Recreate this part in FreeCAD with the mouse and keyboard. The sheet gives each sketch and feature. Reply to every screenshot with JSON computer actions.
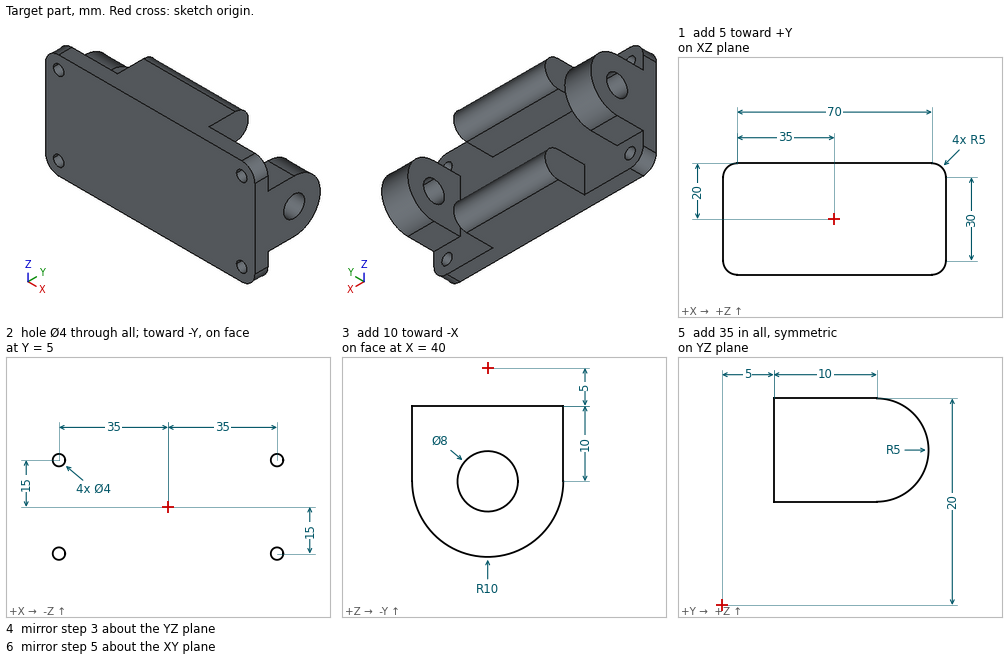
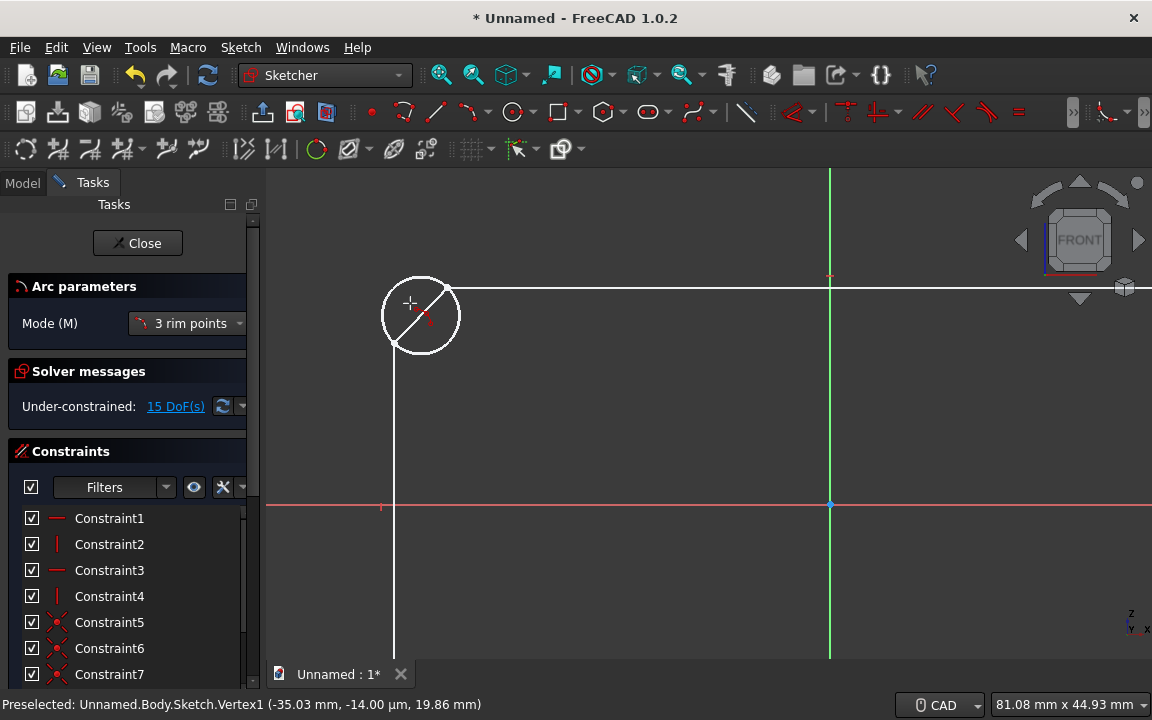
{"action": "left_click", "coordinate": [409, 302]}
{"action": "key", "text": "Escape"}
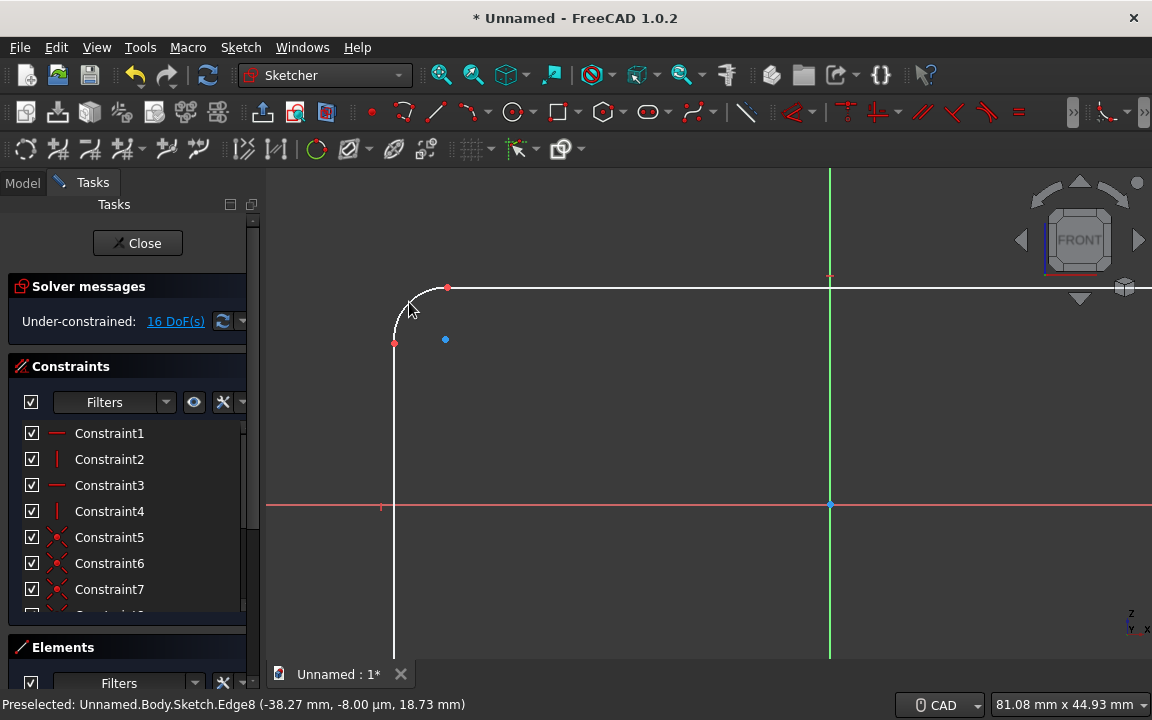
{"action": "left_click", "coordinate": [677, 288]}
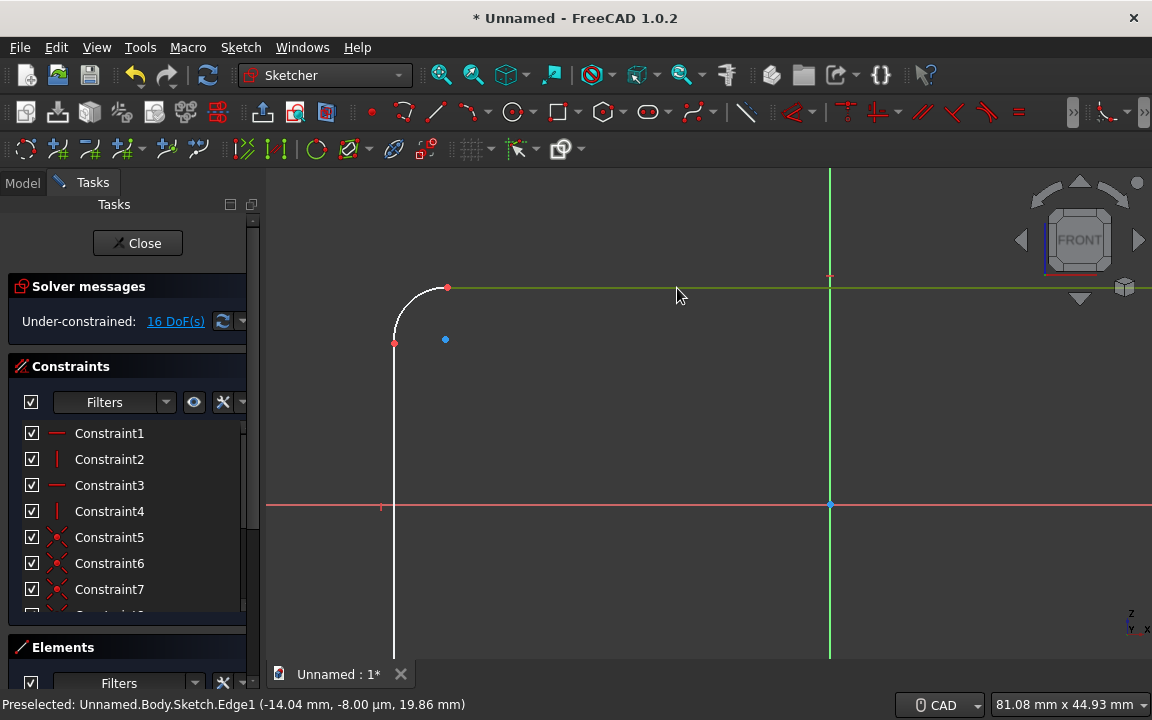
{"action": "scroll", "coordinate": [410, 303], "scroll_direction": "down", "scroll_amount": 3}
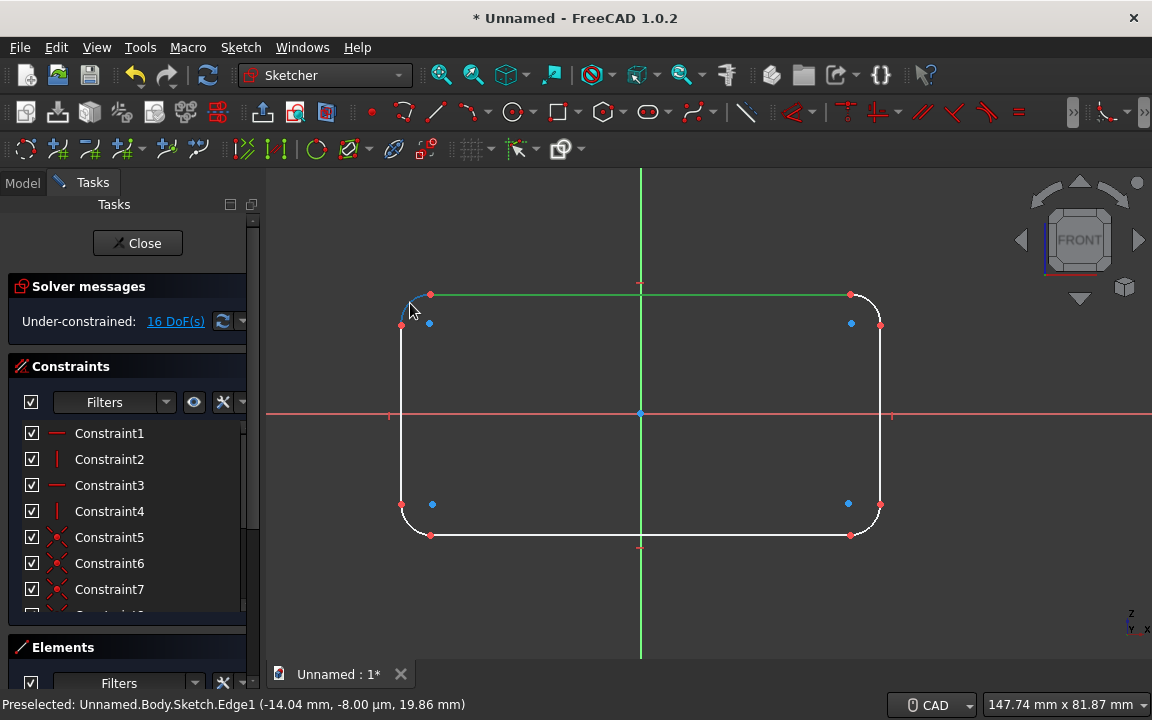
{"action": "left_click", "coordinate": [878, 311]}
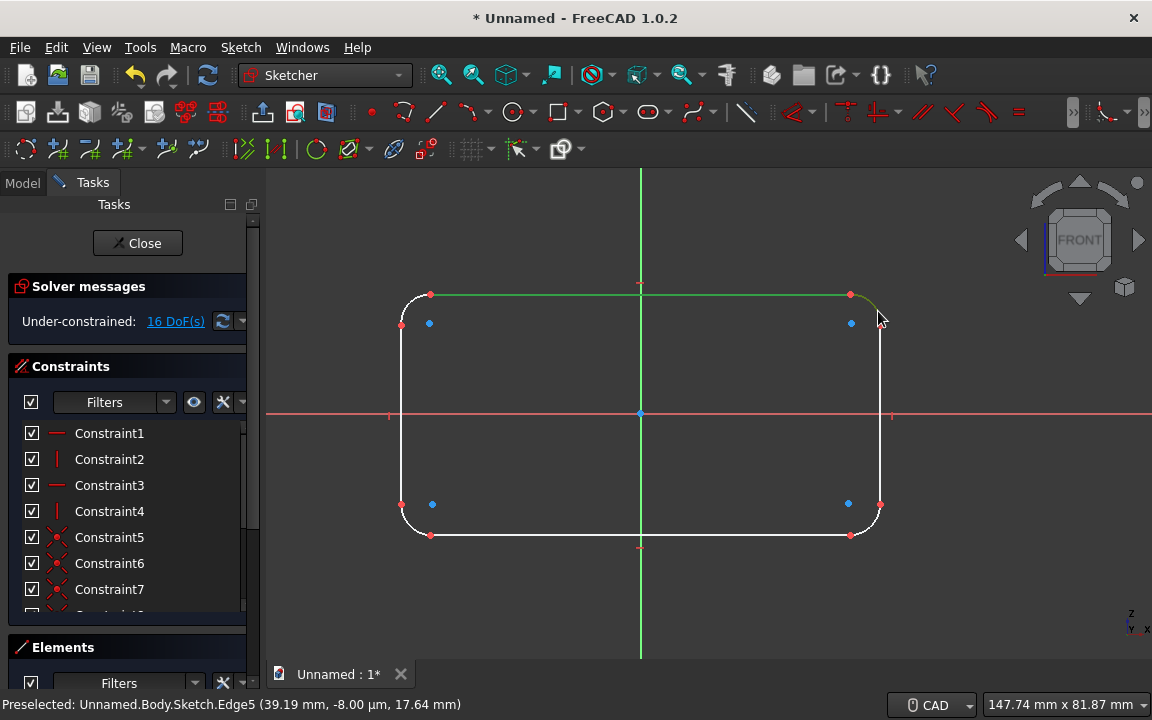
{"action": "key", "text": "t"}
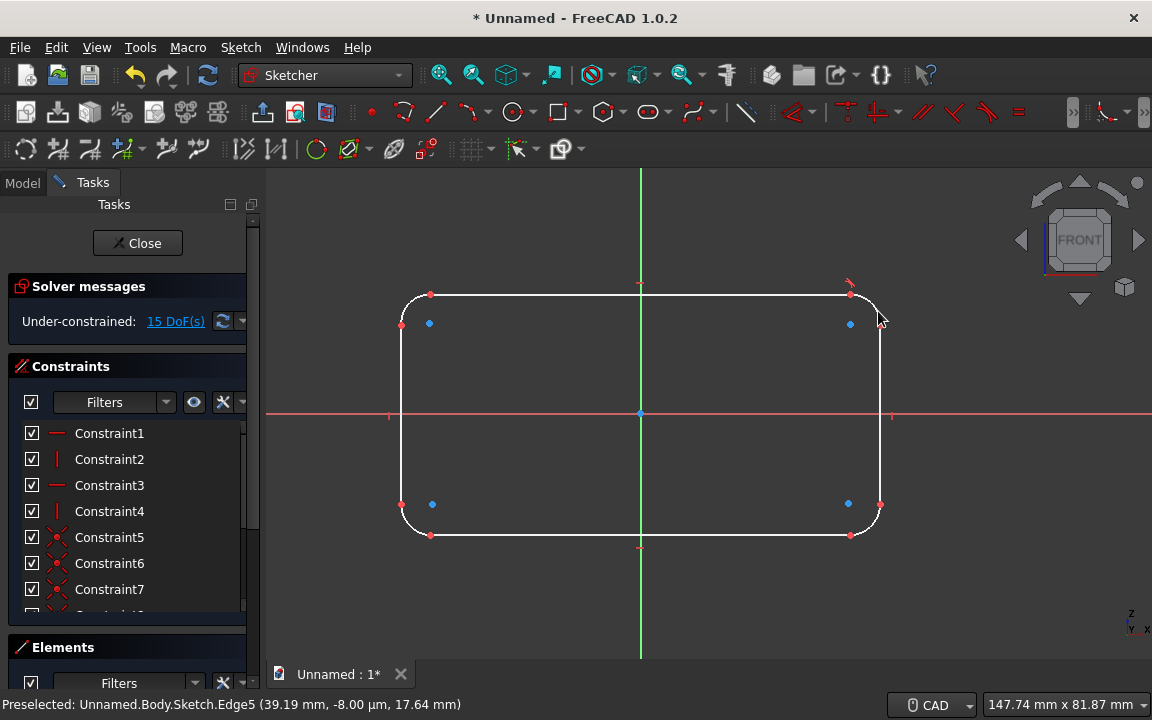
{"action": "left_click", "coordinate": [557, 295]}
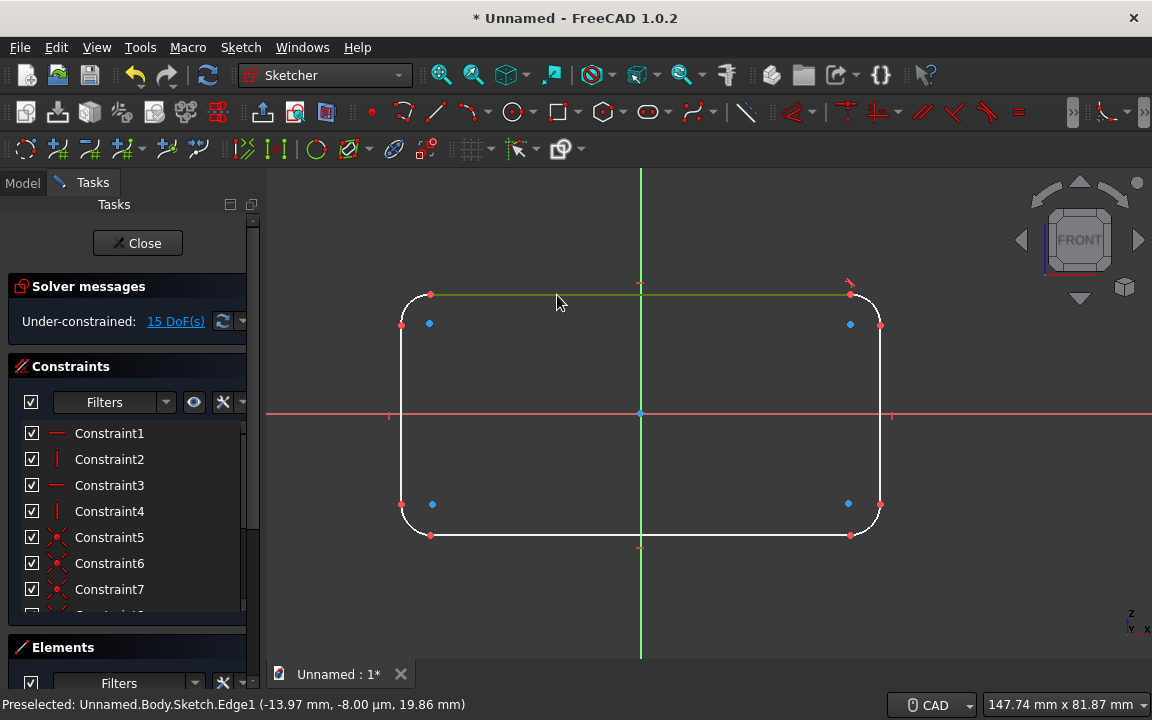
{"action": "left_click", "coordinate": [417, 298]}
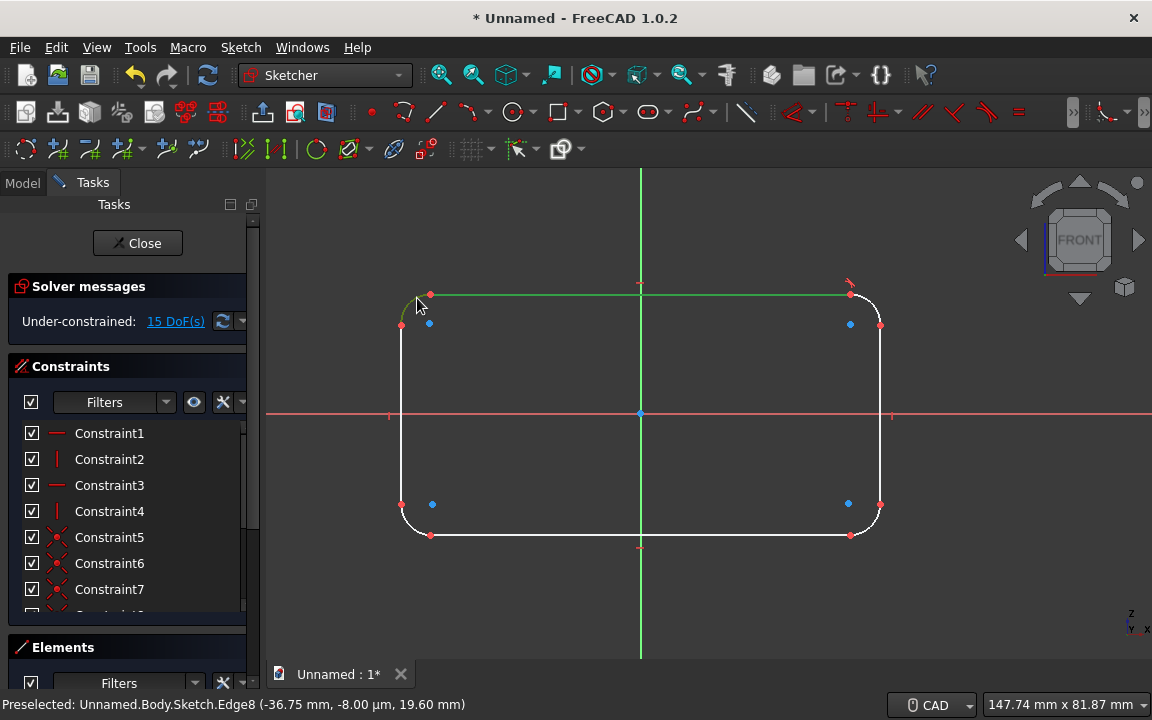
{"action": "key", "text": "t"}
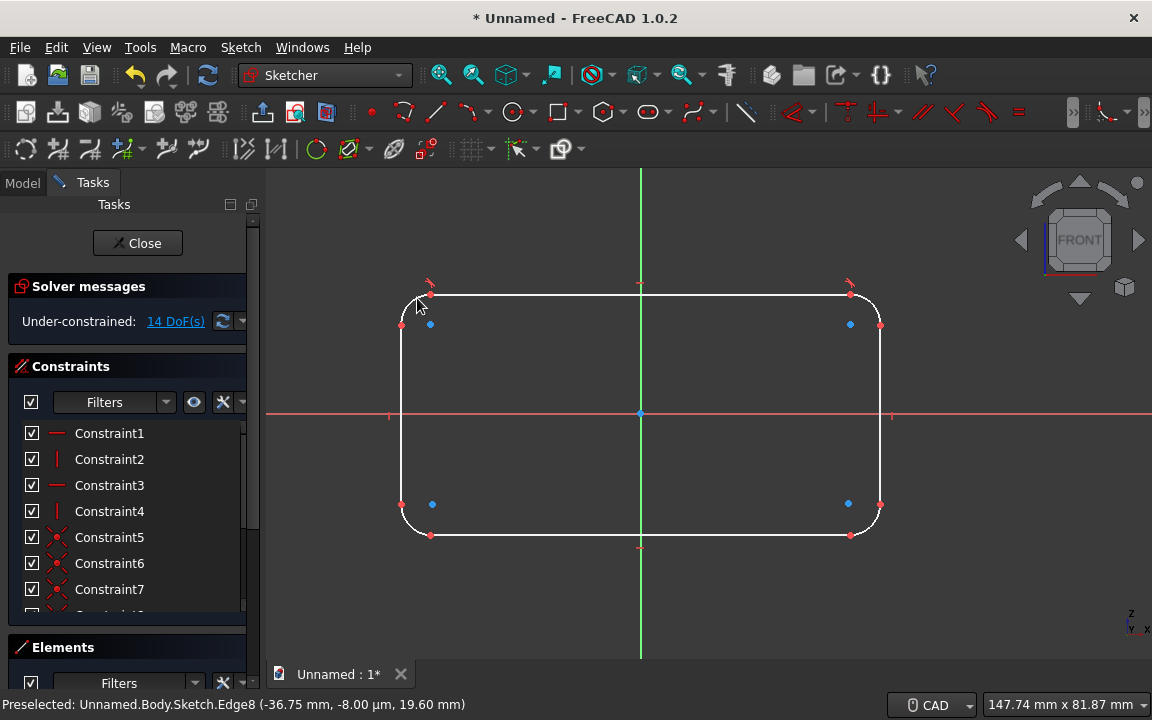
{"action": "left_click", "coordinate": [880, 379]}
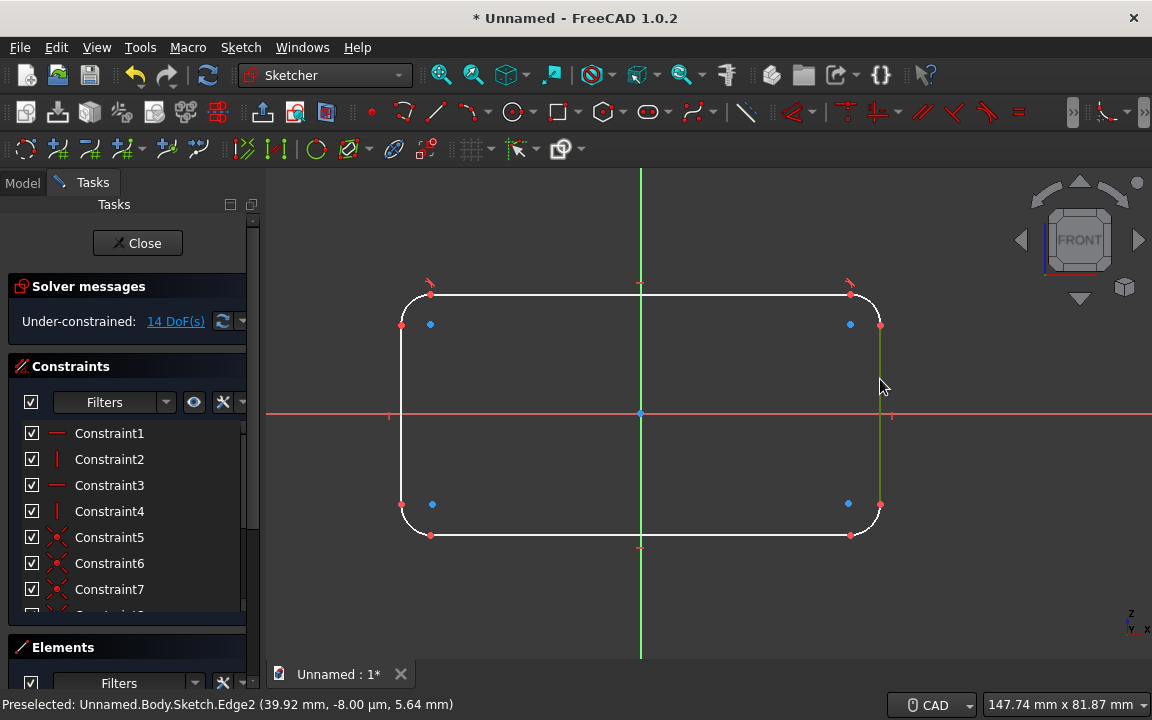
{"action": "left_click", "coordinate": [877, 311]}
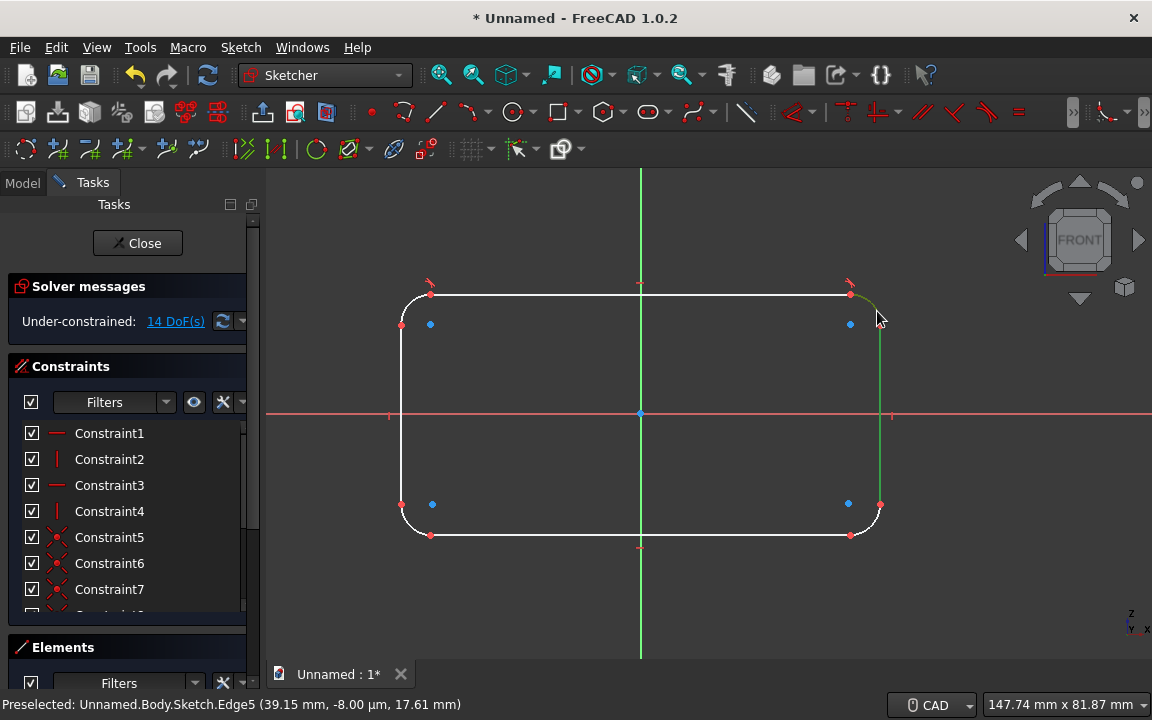
{"action": "key", "text": "t"}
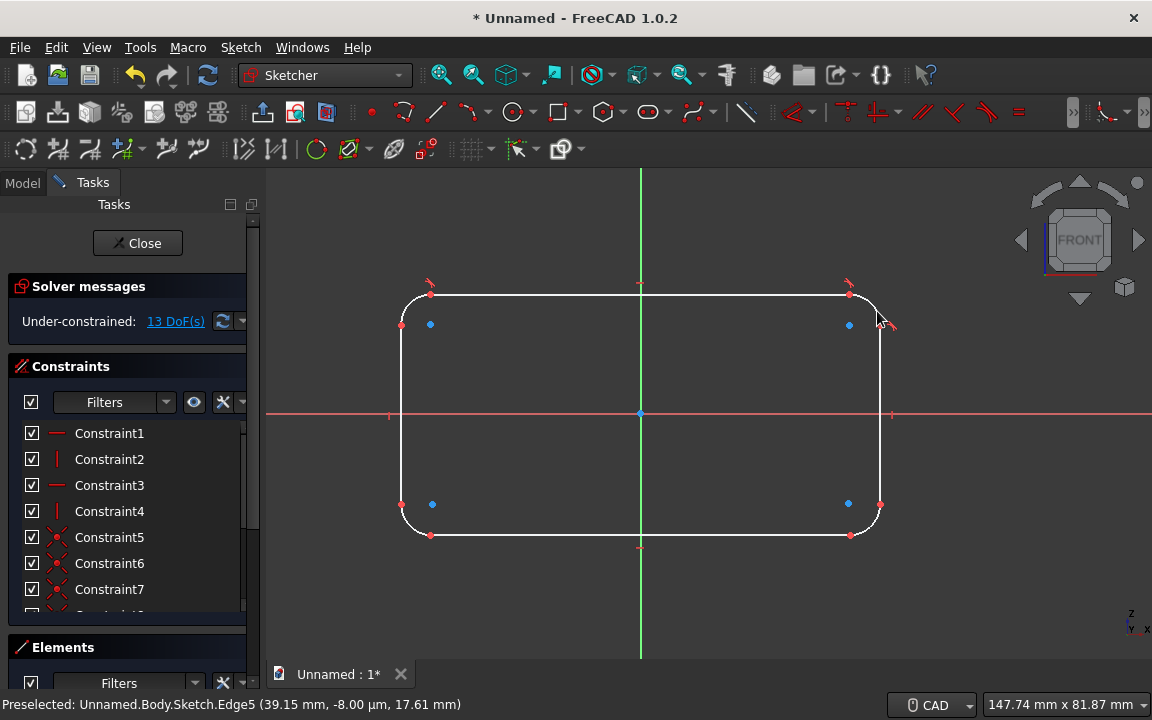
{"action": "left_click", "coordinate": [880, 379]}